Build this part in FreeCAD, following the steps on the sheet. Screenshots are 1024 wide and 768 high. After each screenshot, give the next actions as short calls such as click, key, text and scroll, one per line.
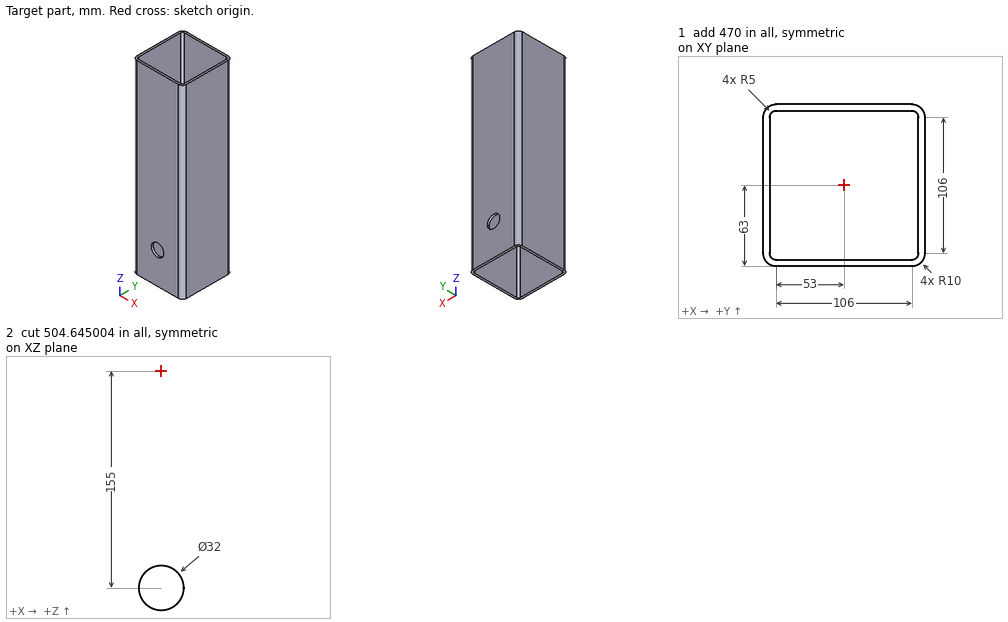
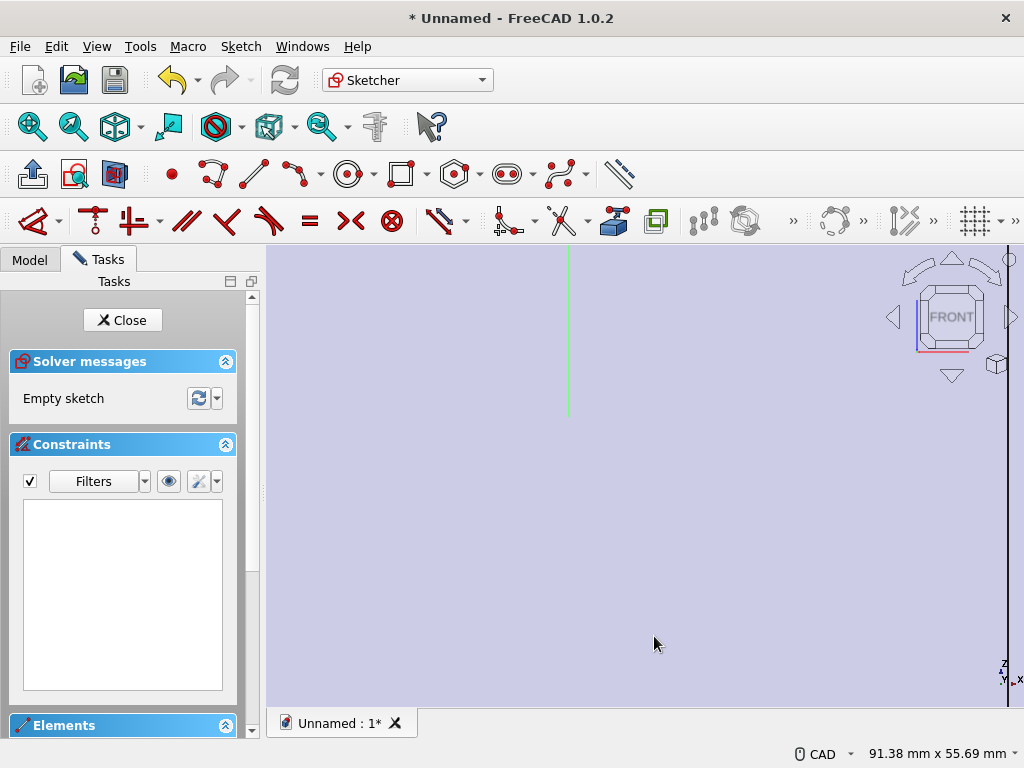
click(348, 174)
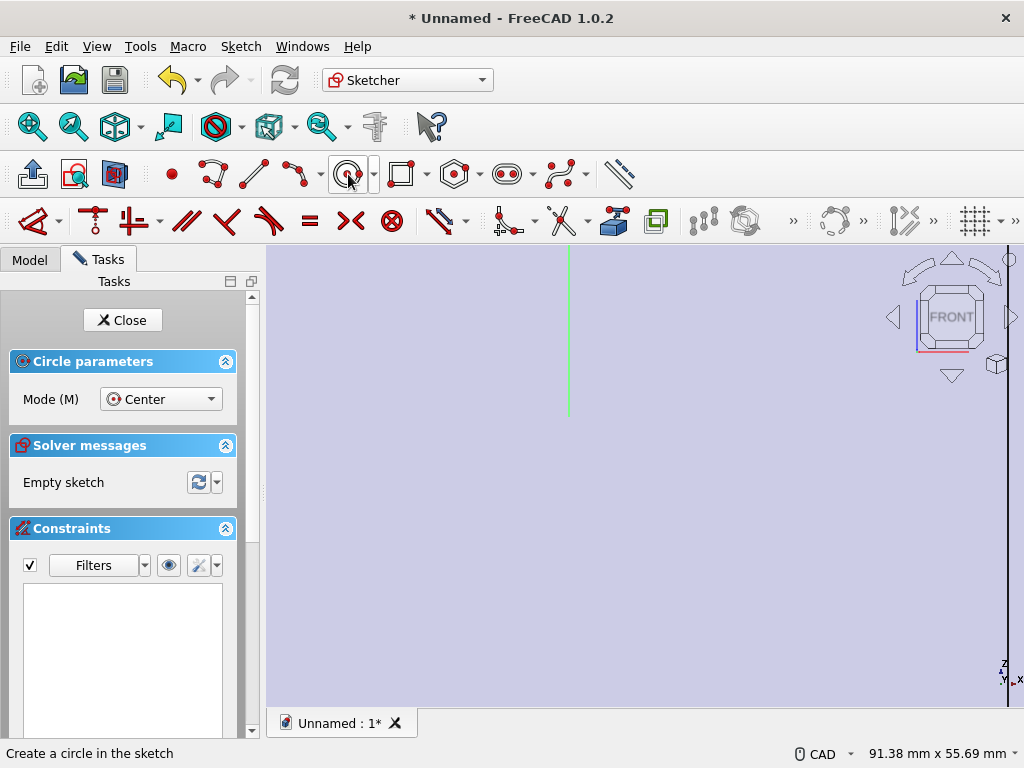
click(569, 471)
move(663, 377)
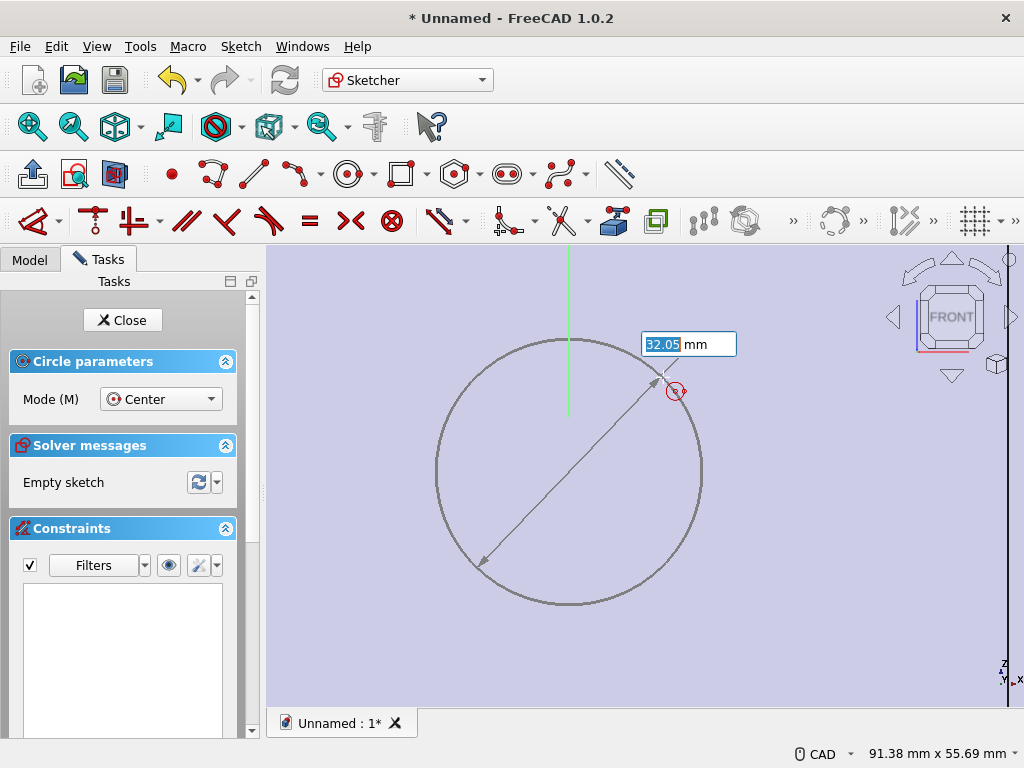
text(32)
key(Return)
key(Escape)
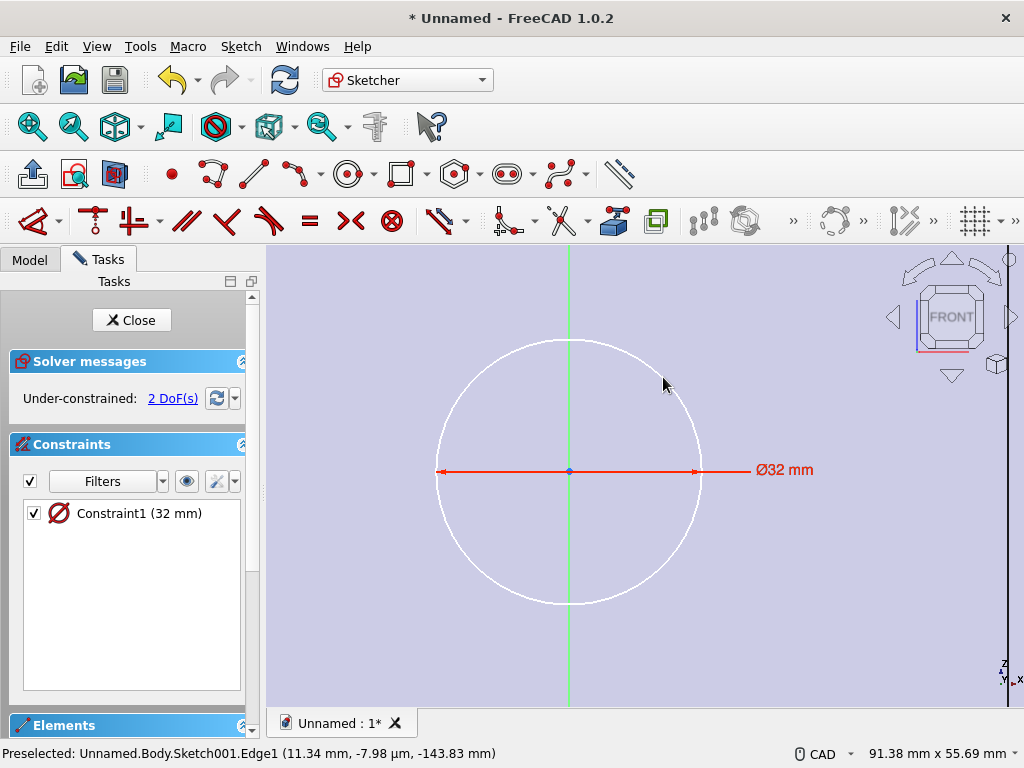
click(569, 472)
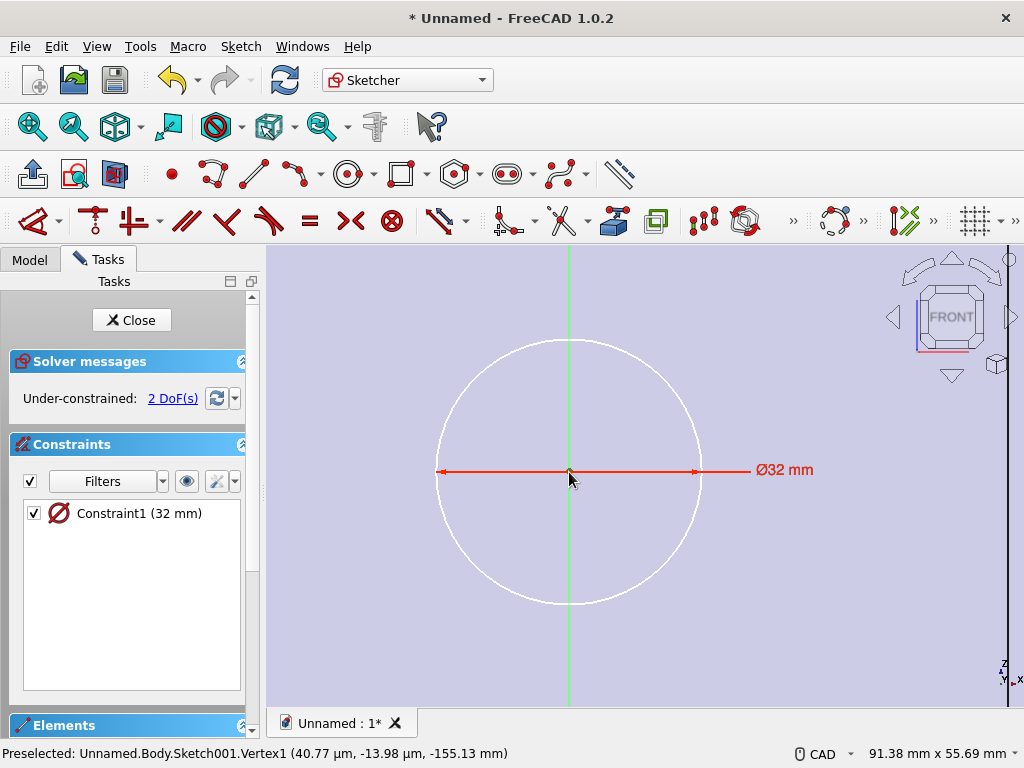
click(569, 650)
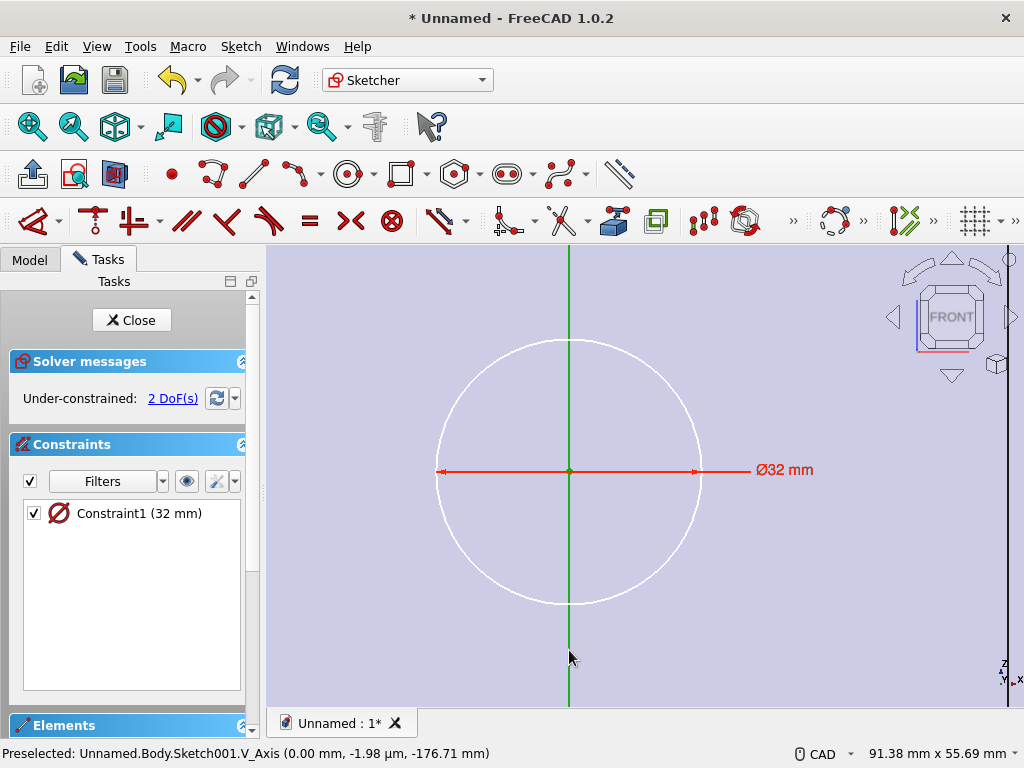
click(93, 222)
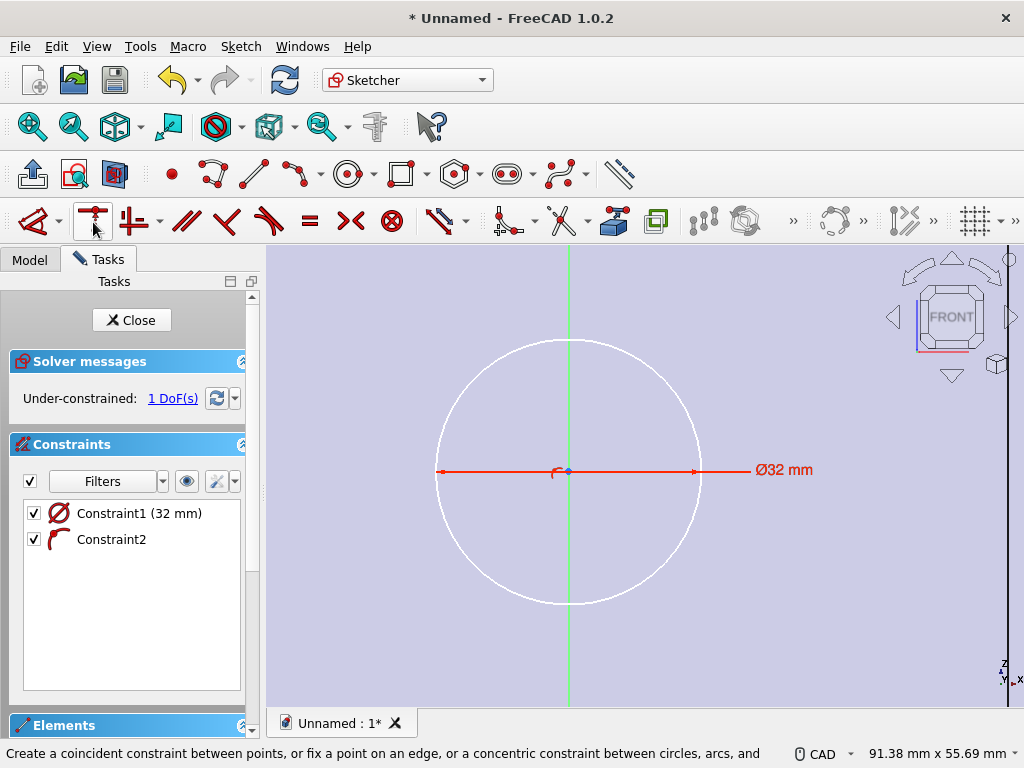
click(32, 222)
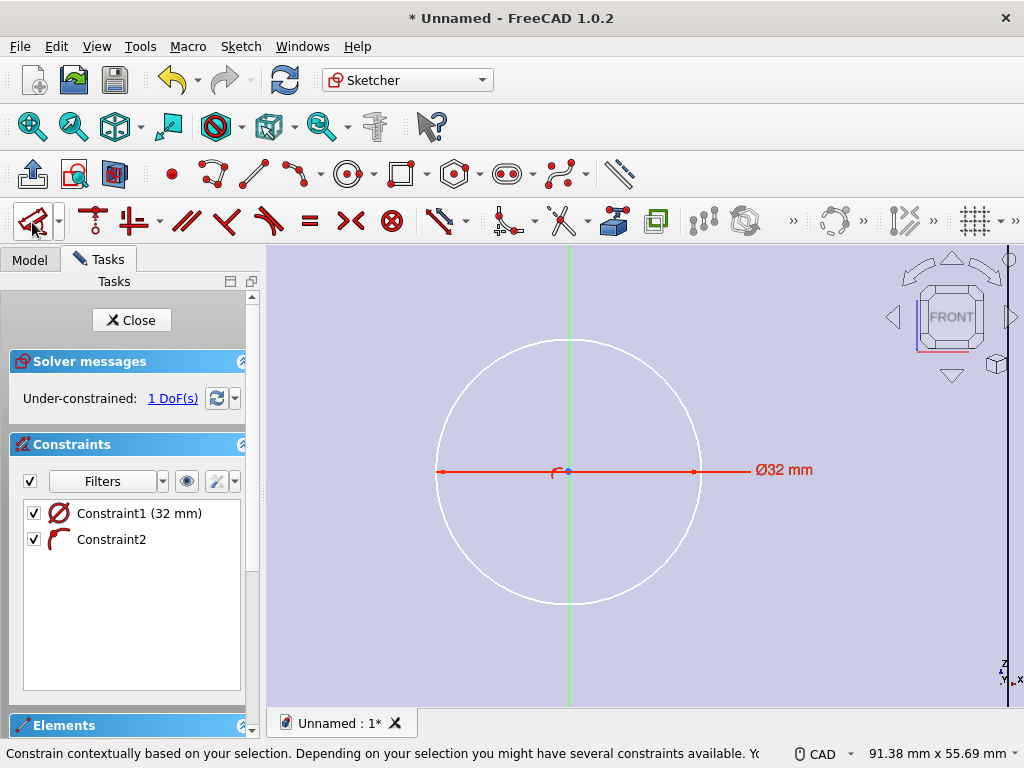
click(569, 472)
click(603, 372)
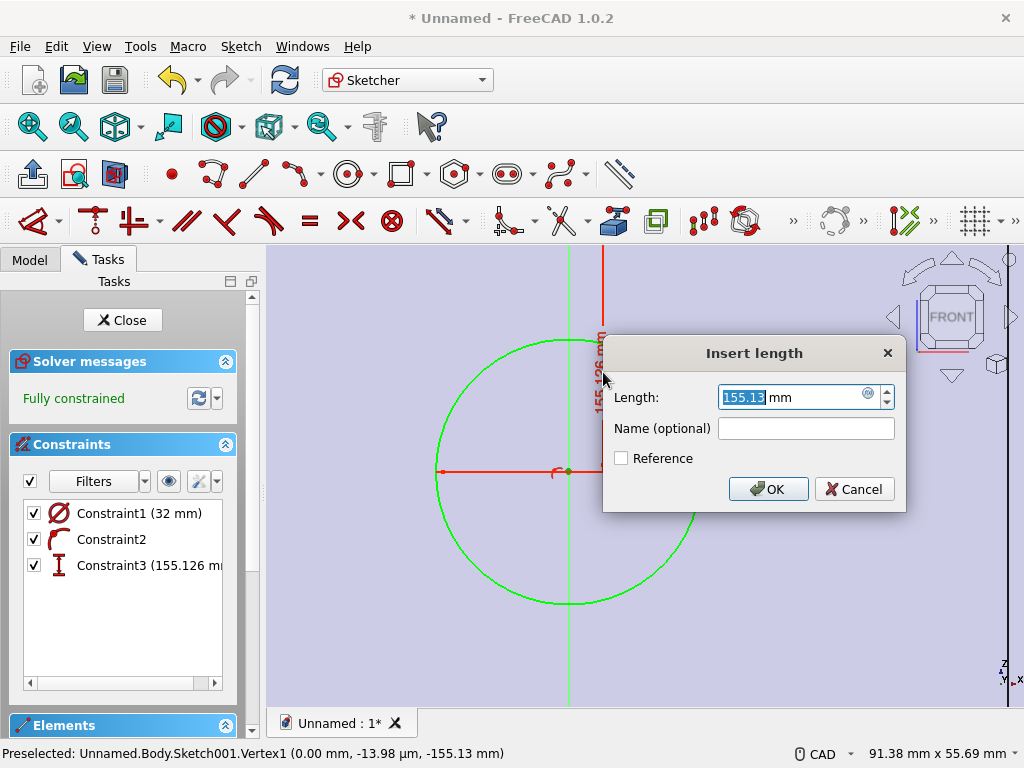
text(155)
key(Return)
key(Escape)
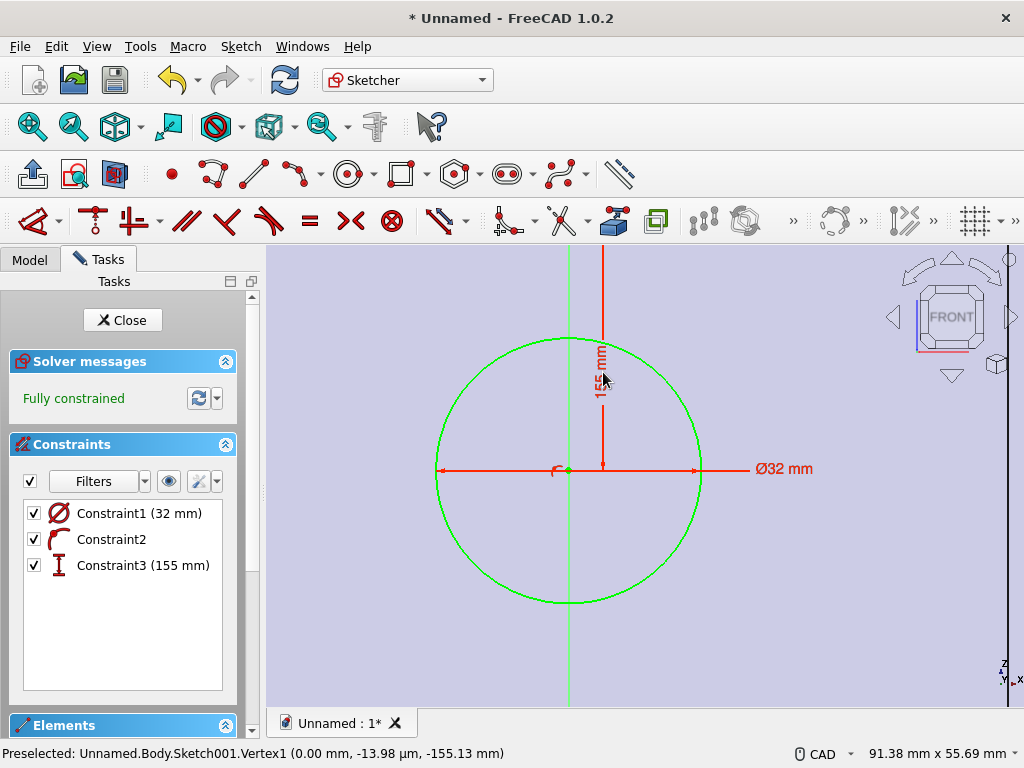
click(123, 320)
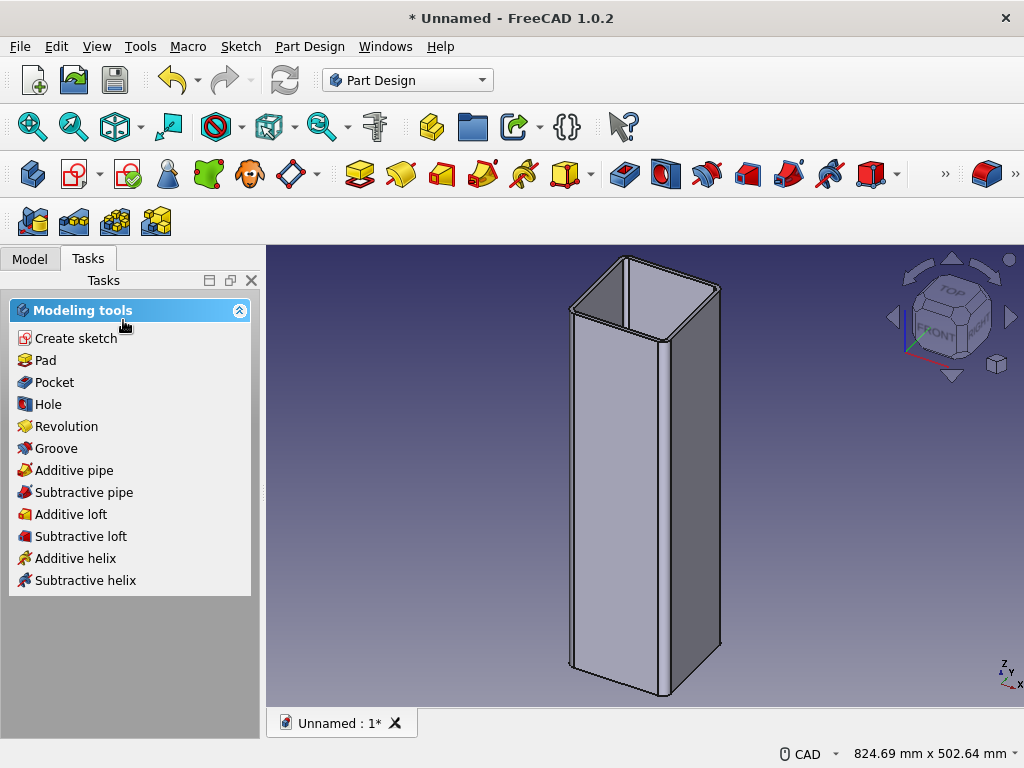
click(625, 174)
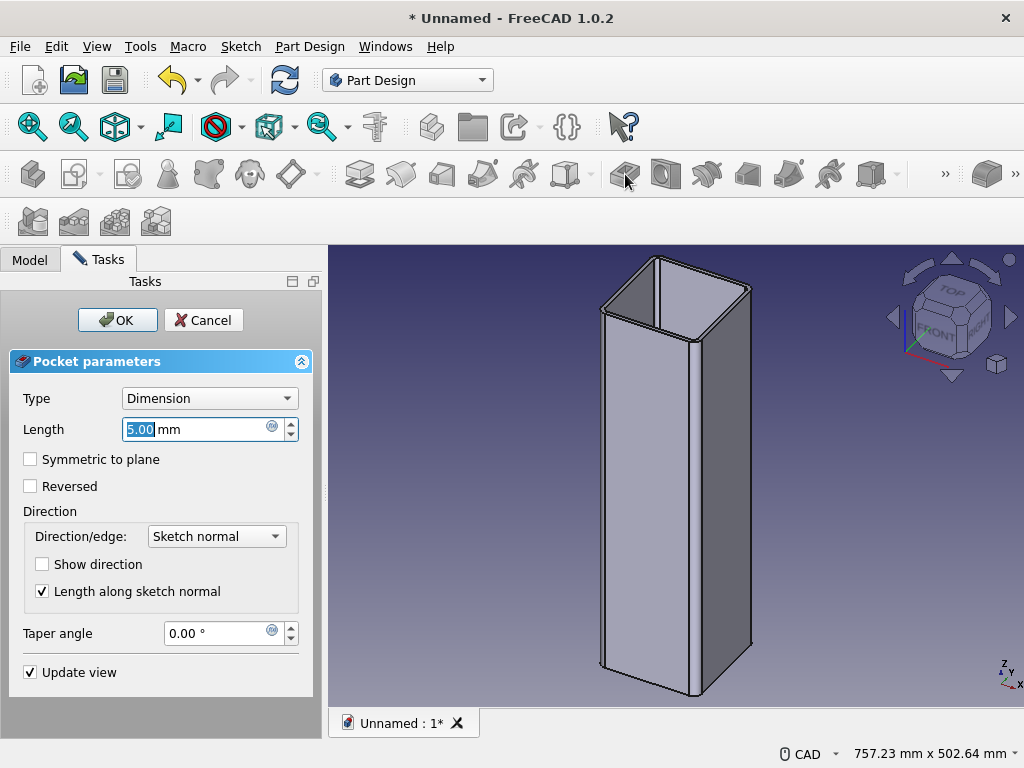
text(504.645004)
key(Tab)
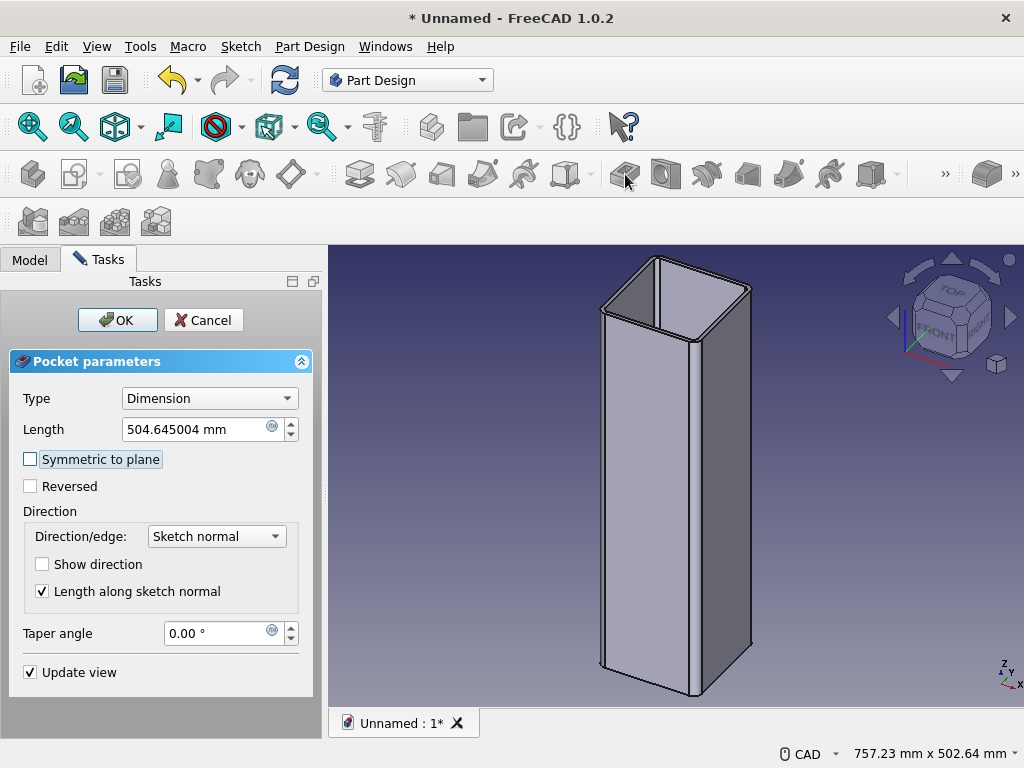
click(31, 459)